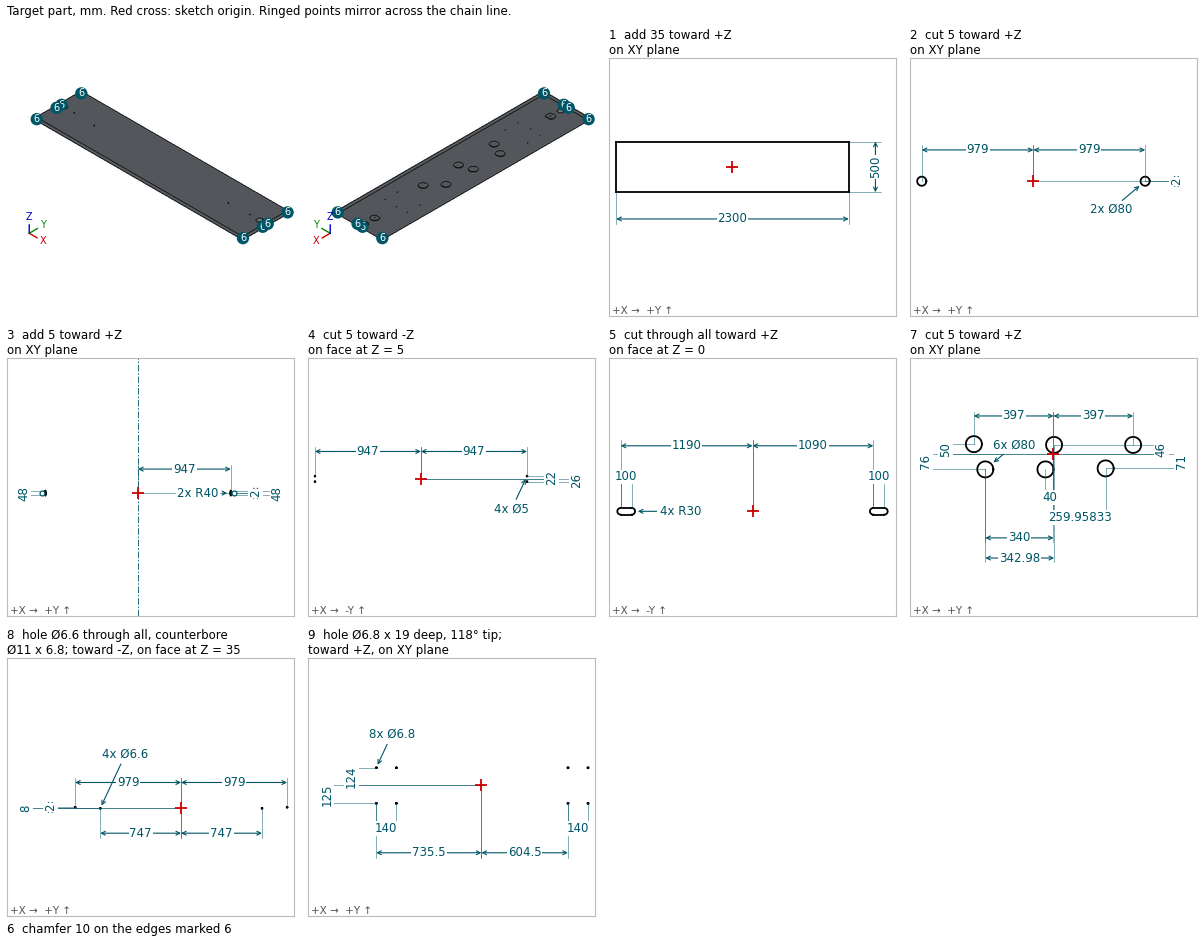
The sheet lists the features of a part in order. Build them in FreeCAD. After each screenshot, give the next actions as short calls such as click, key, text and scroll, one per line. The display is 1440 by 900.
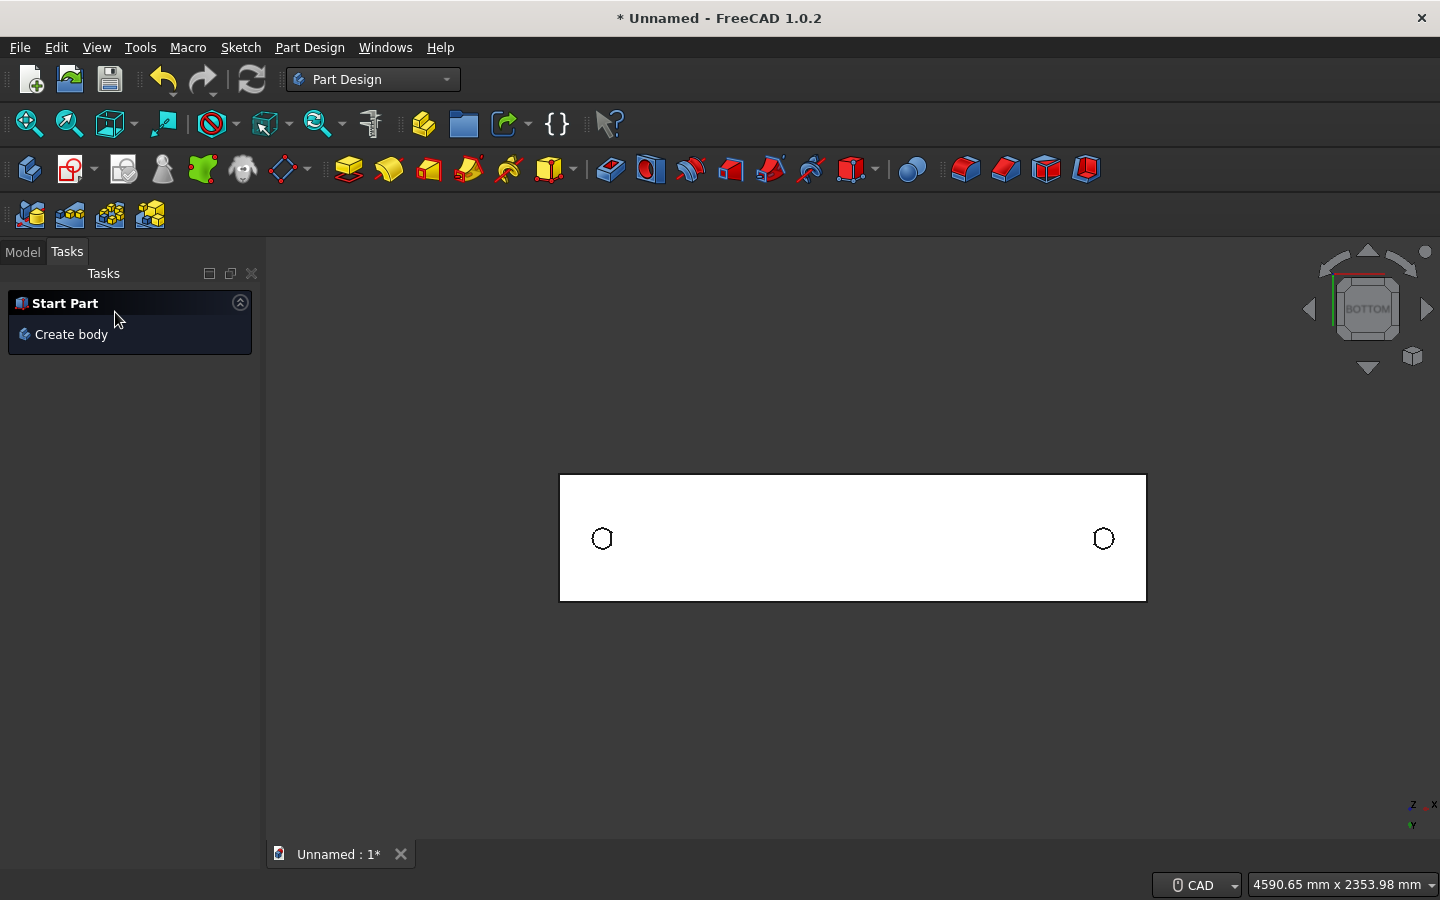
click(1021, 537)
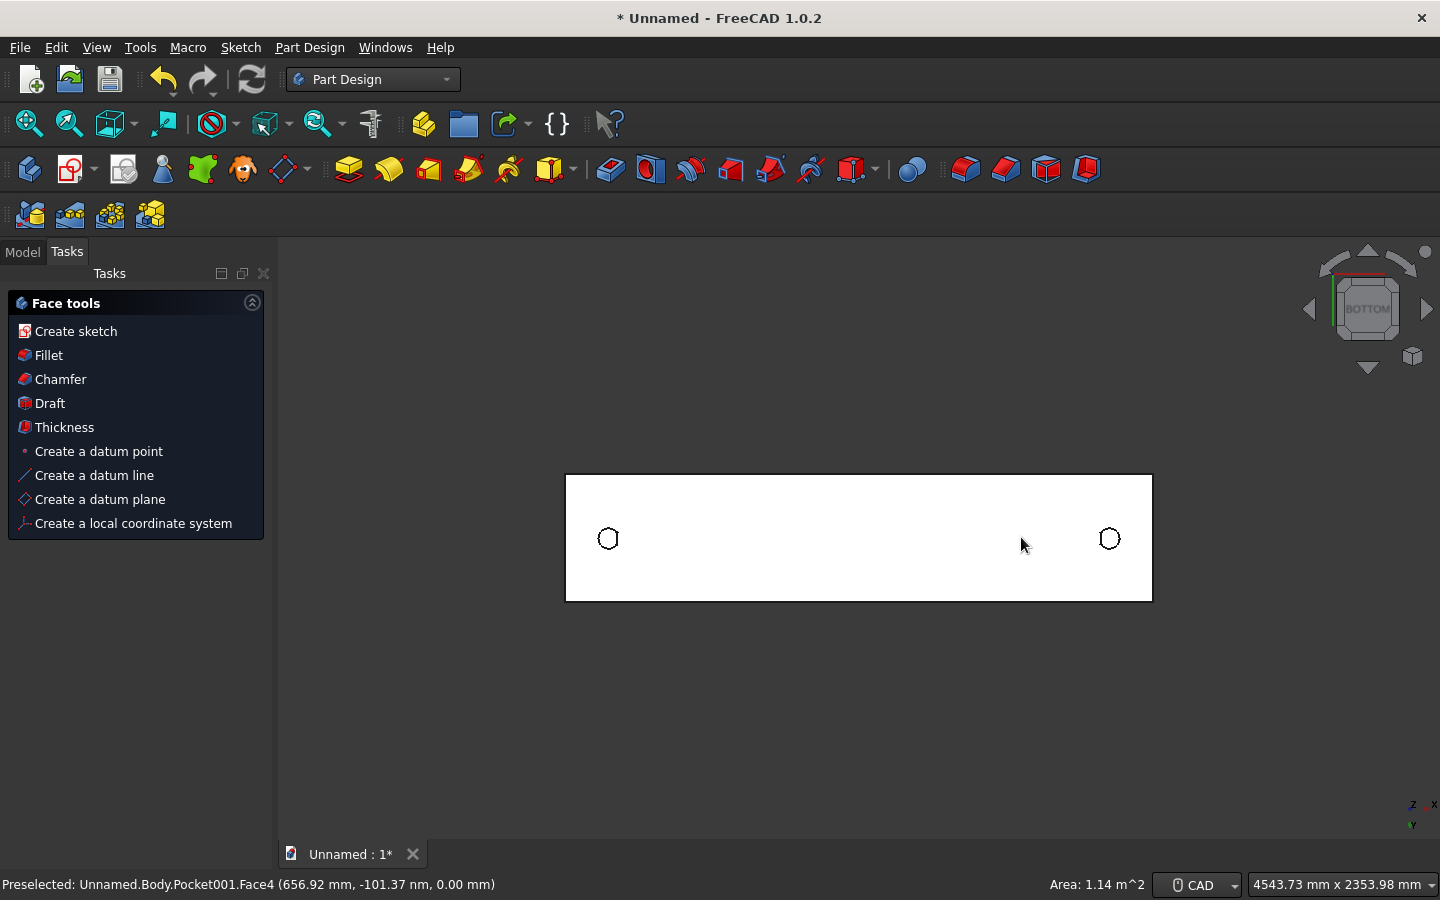
click(70, 170)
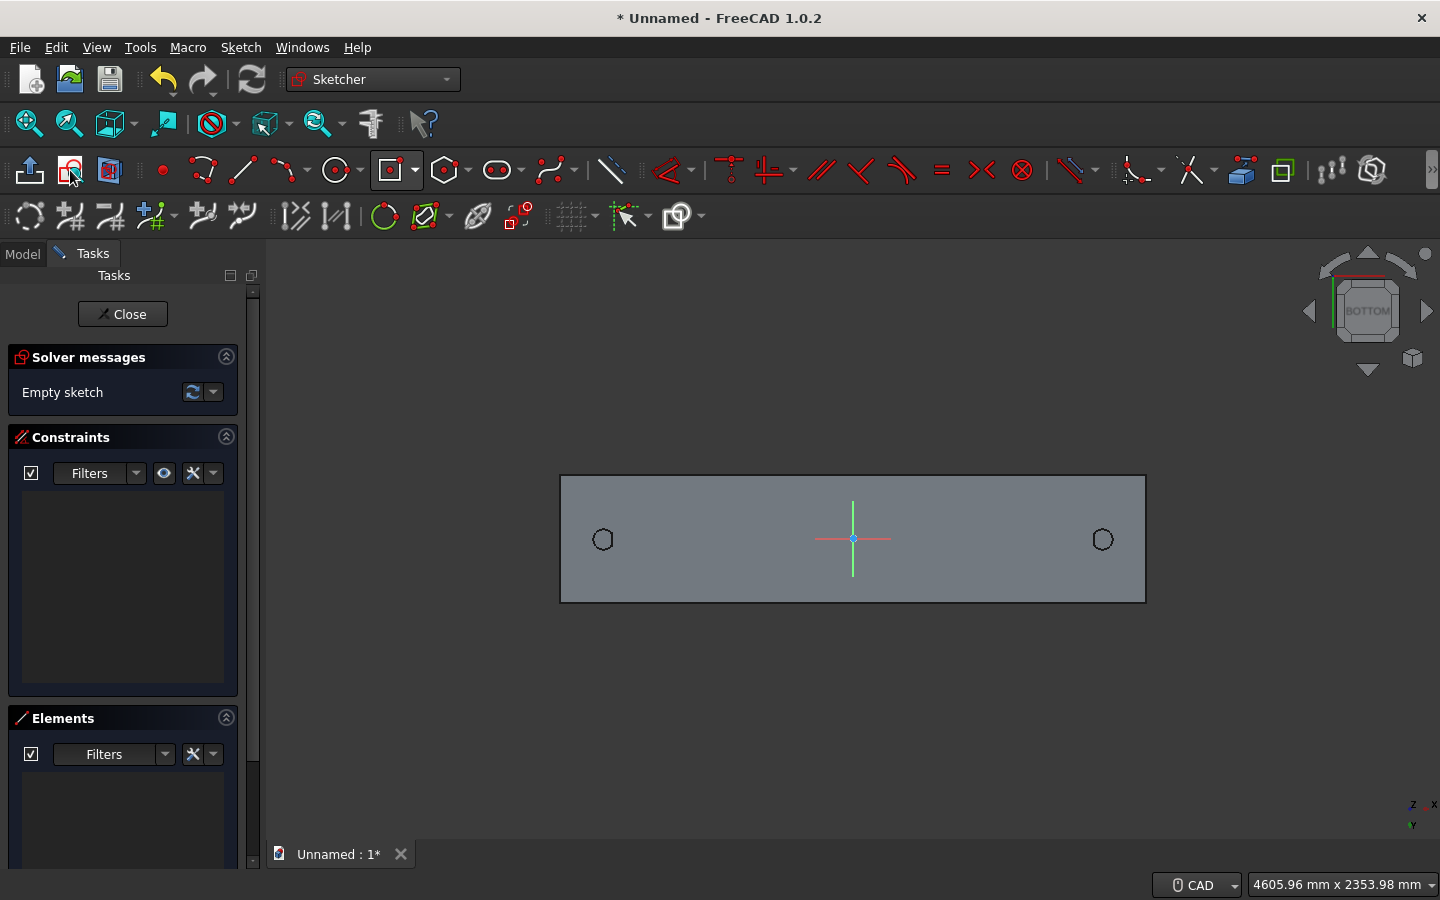
click(498, 170)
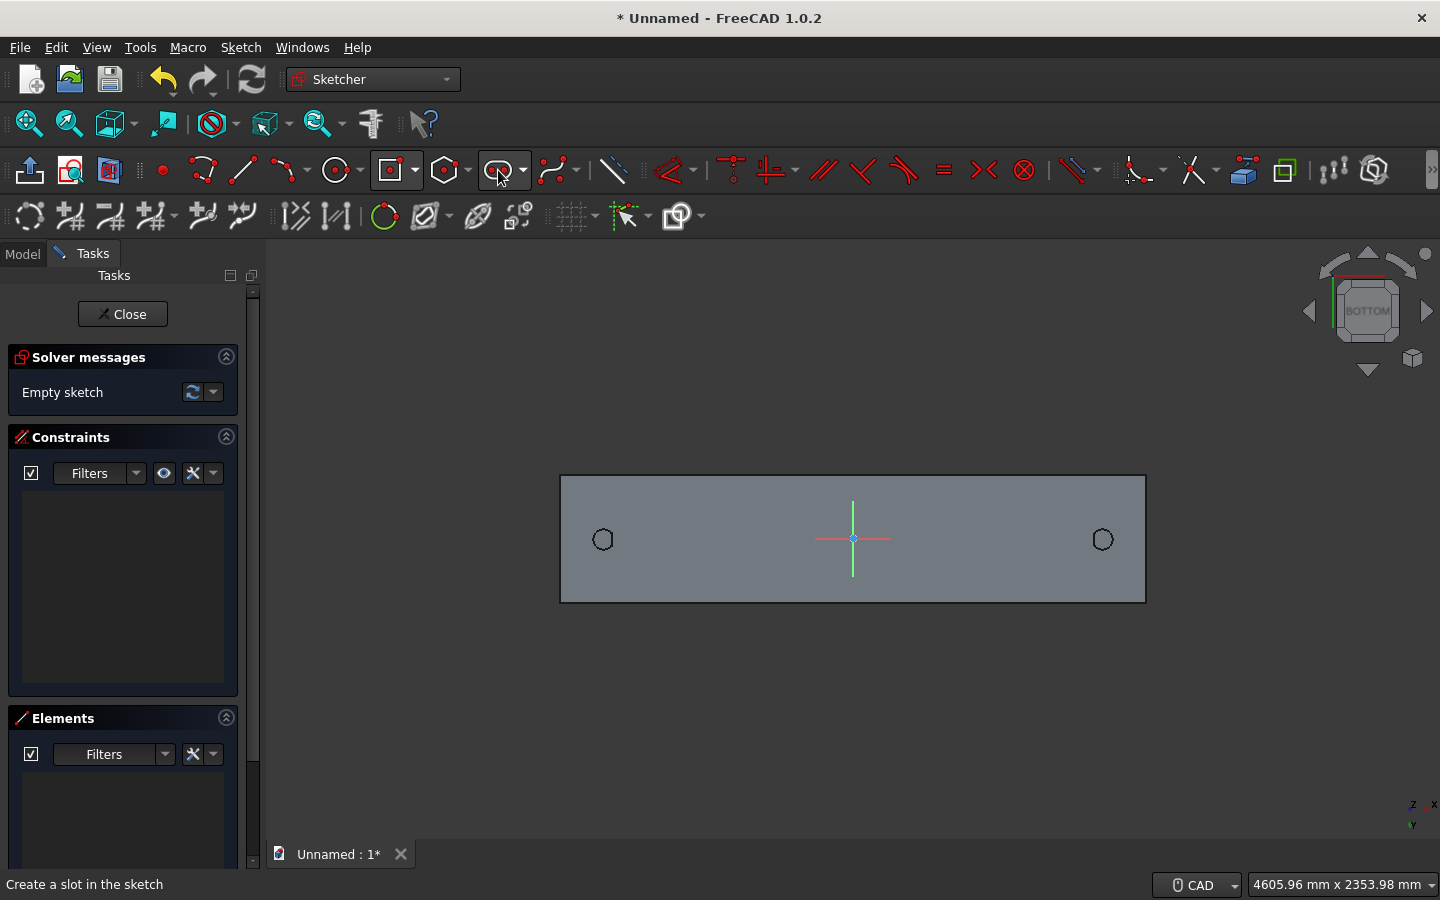
scroll(550, 539, up, 6)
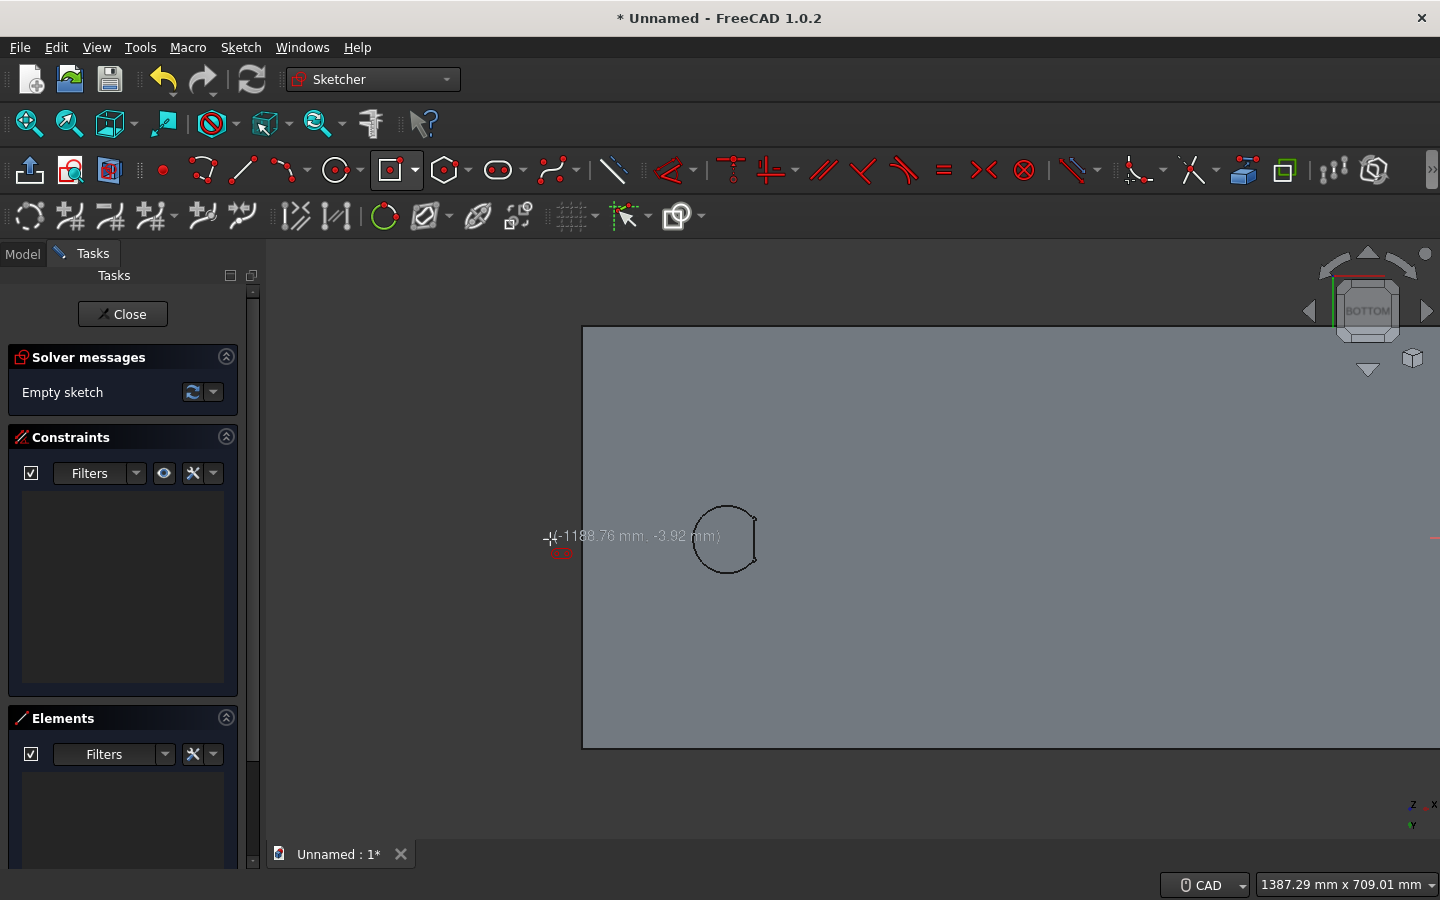
click(548, 538)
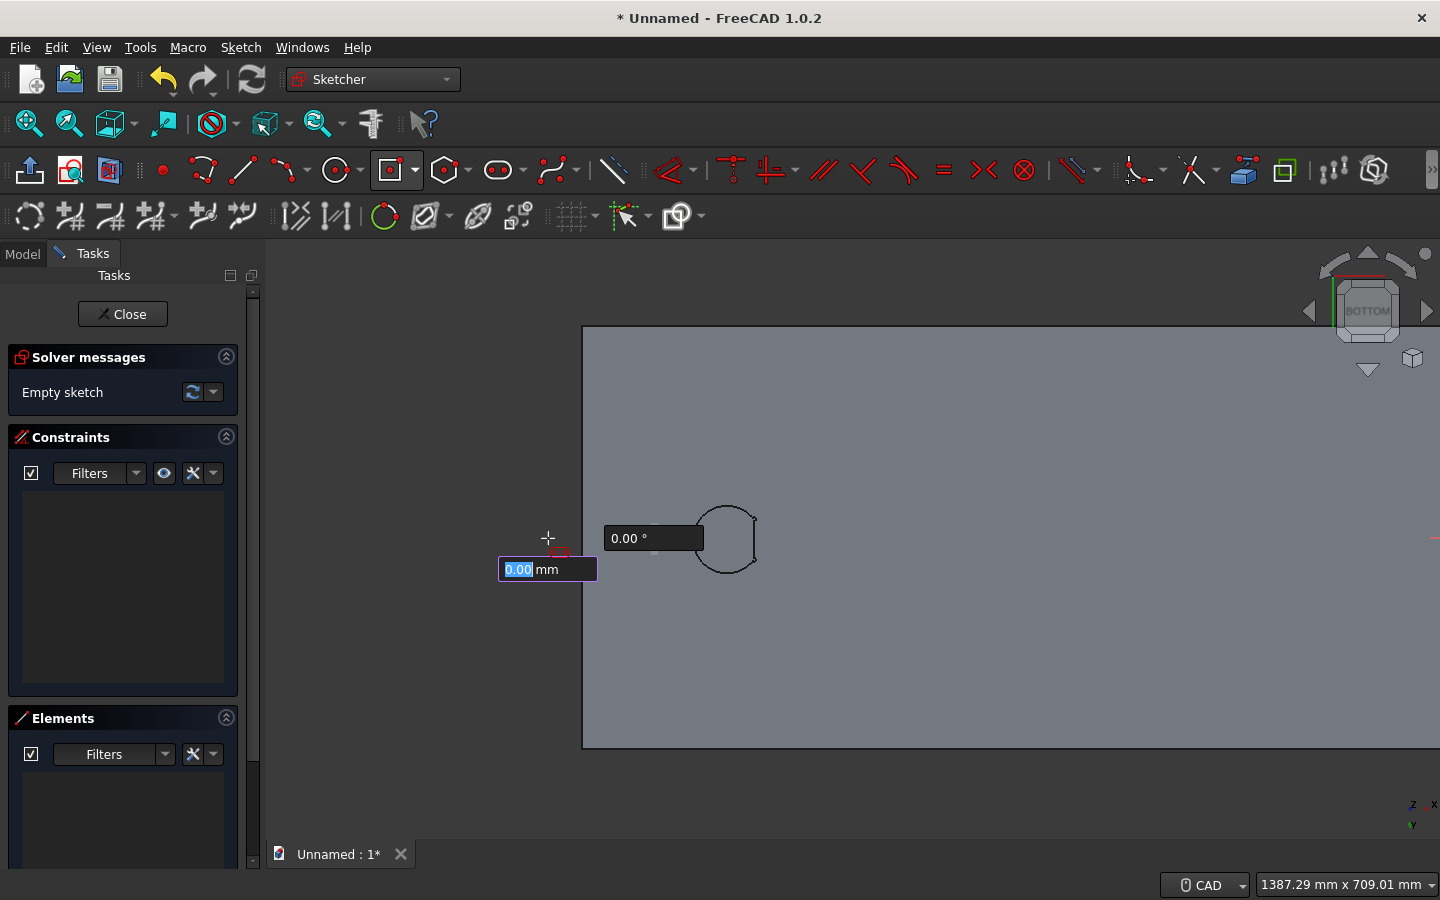
click(633, 529)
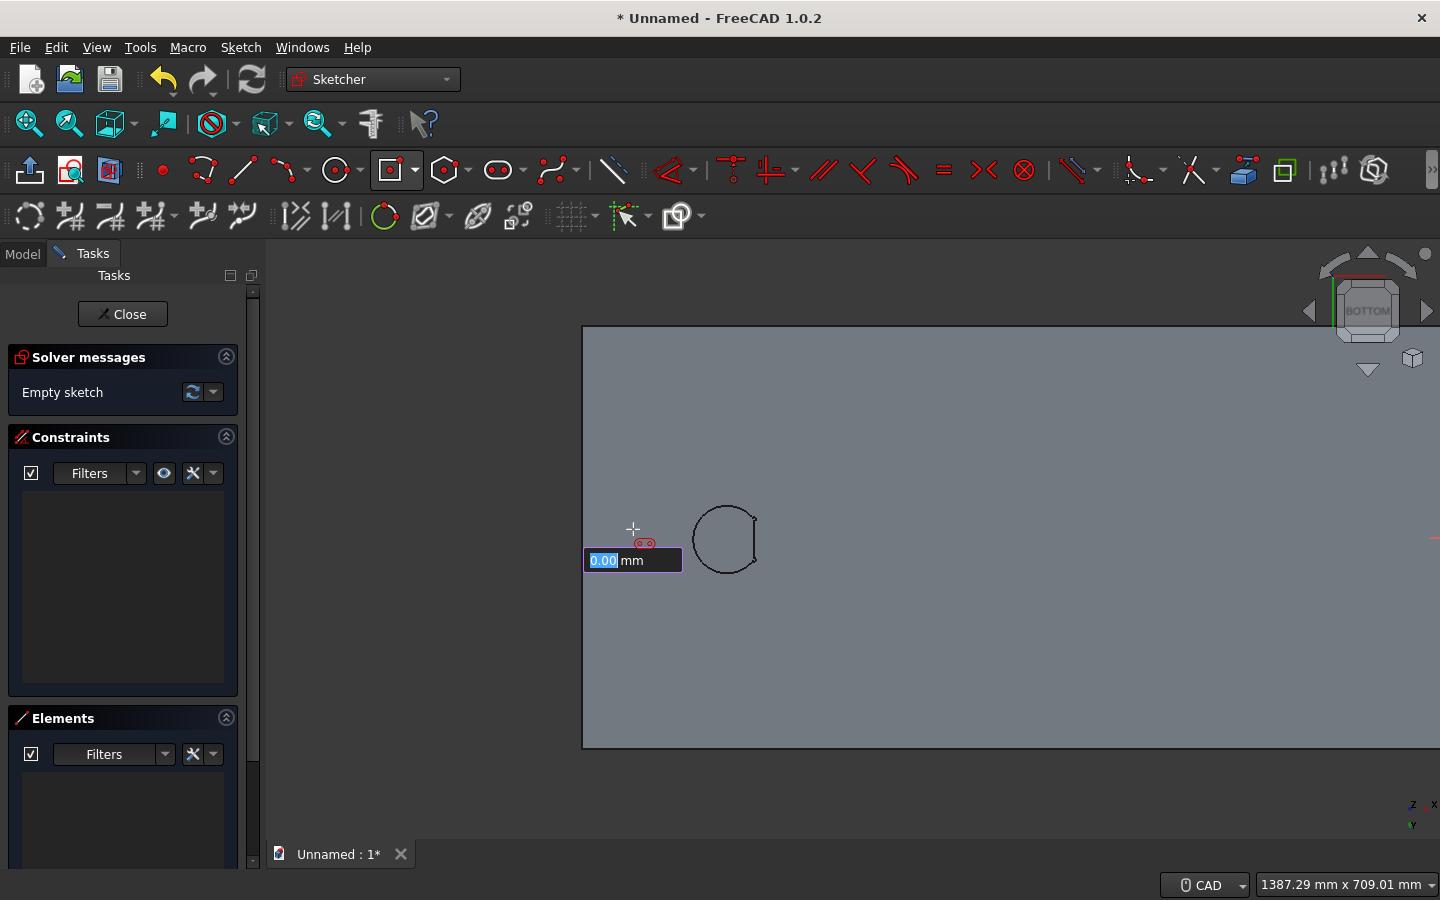
click(591, 563)